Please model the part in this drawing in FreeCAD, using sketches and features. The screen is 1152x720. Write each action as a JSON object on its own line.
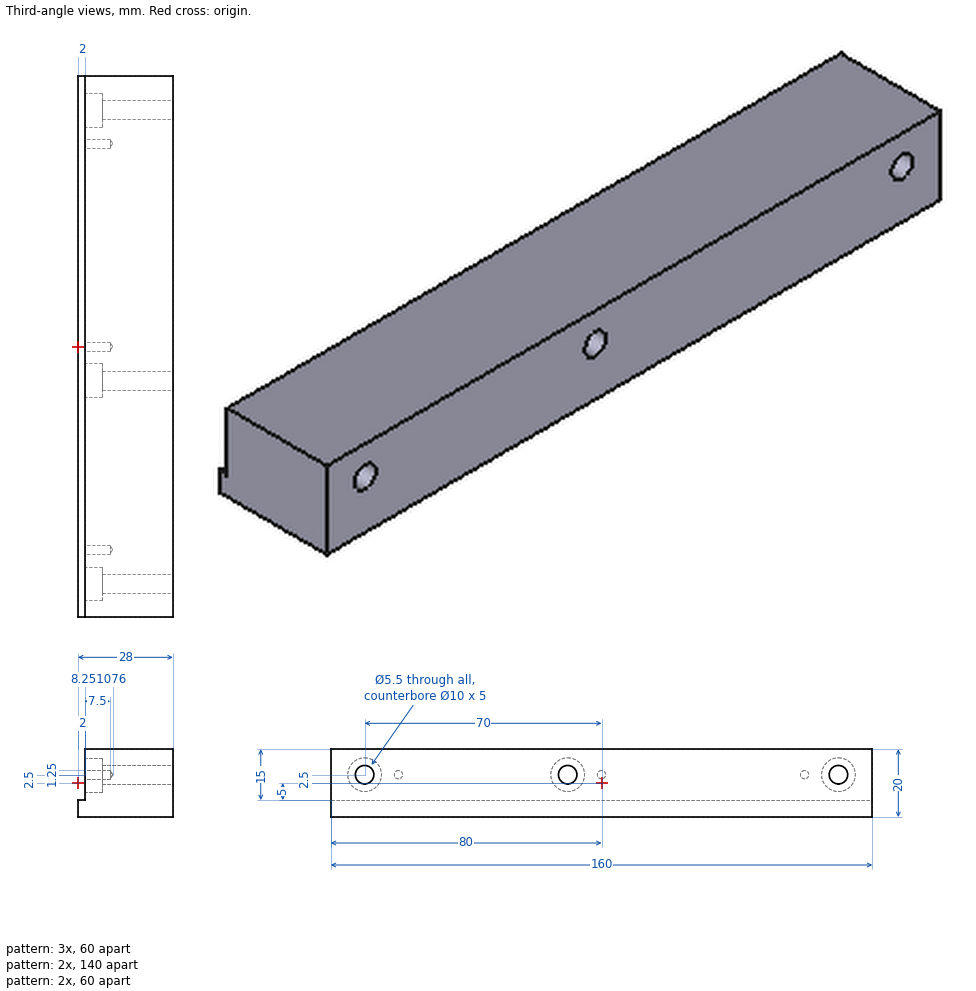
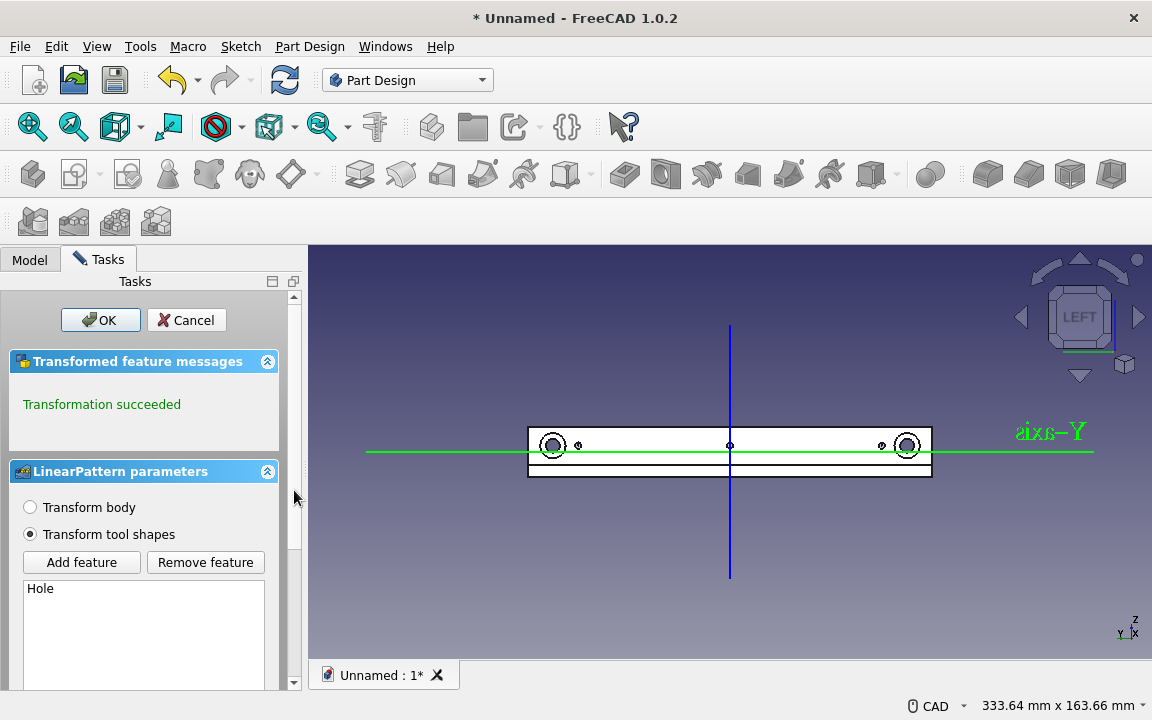
{"action": "left_click", "coordinate": [101, 320]}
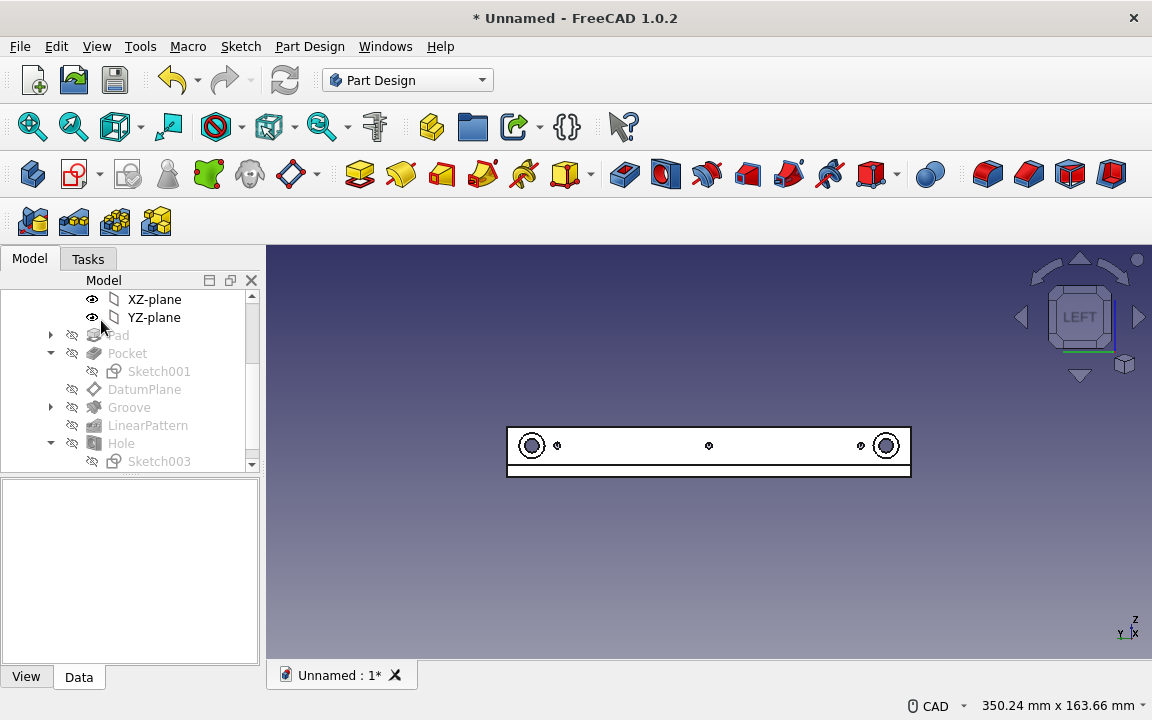
{"action": "left_click", "coordinate": [117, 443]}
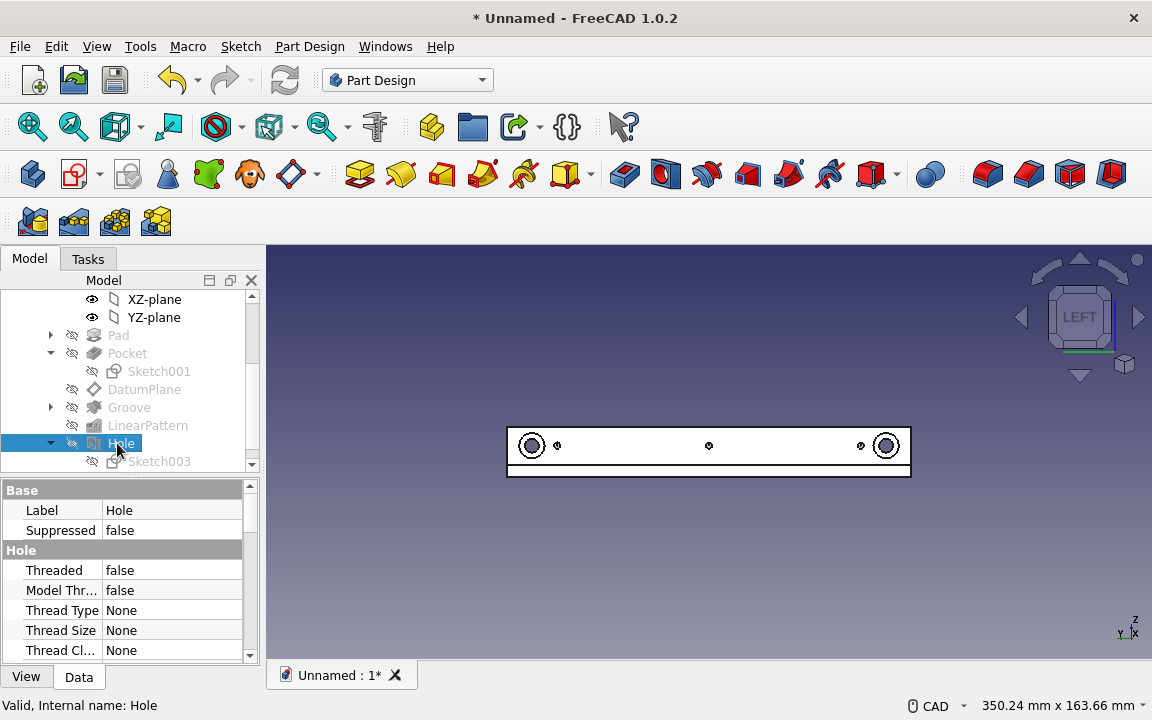
{"action": "left_click", "coordinate": [74, 222]}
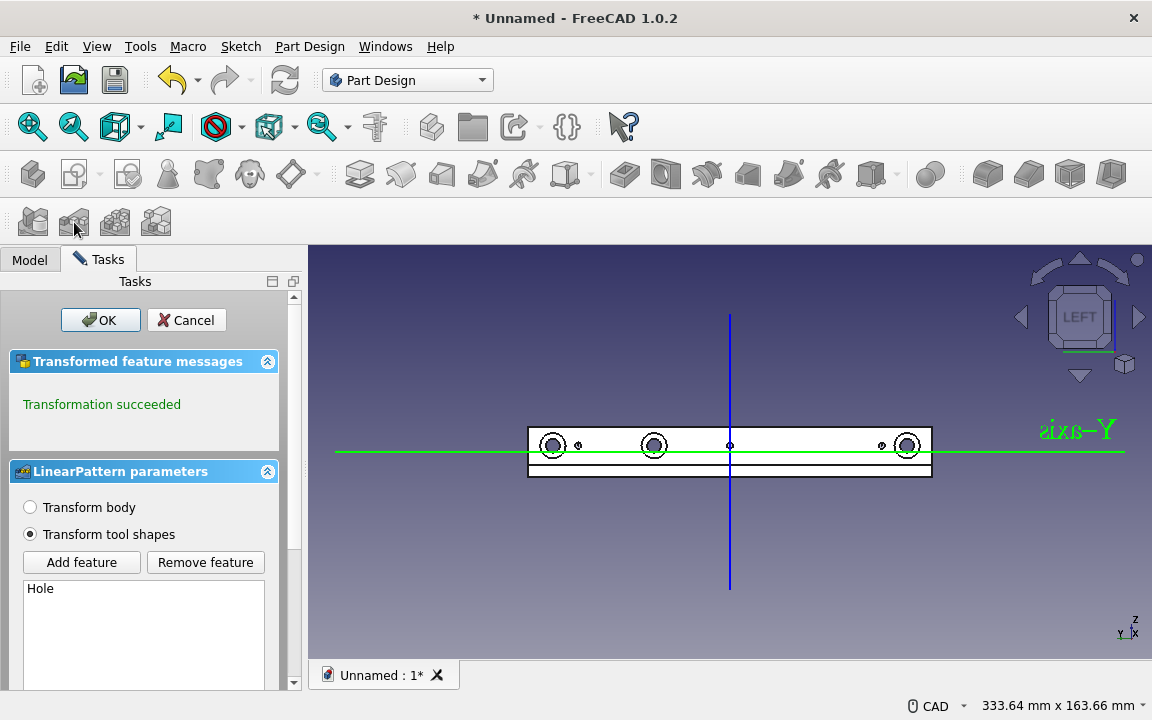
{"action": "scroll", "coordinate": [294, 490], "scroll_direction": "down", "scroll_amount": 2}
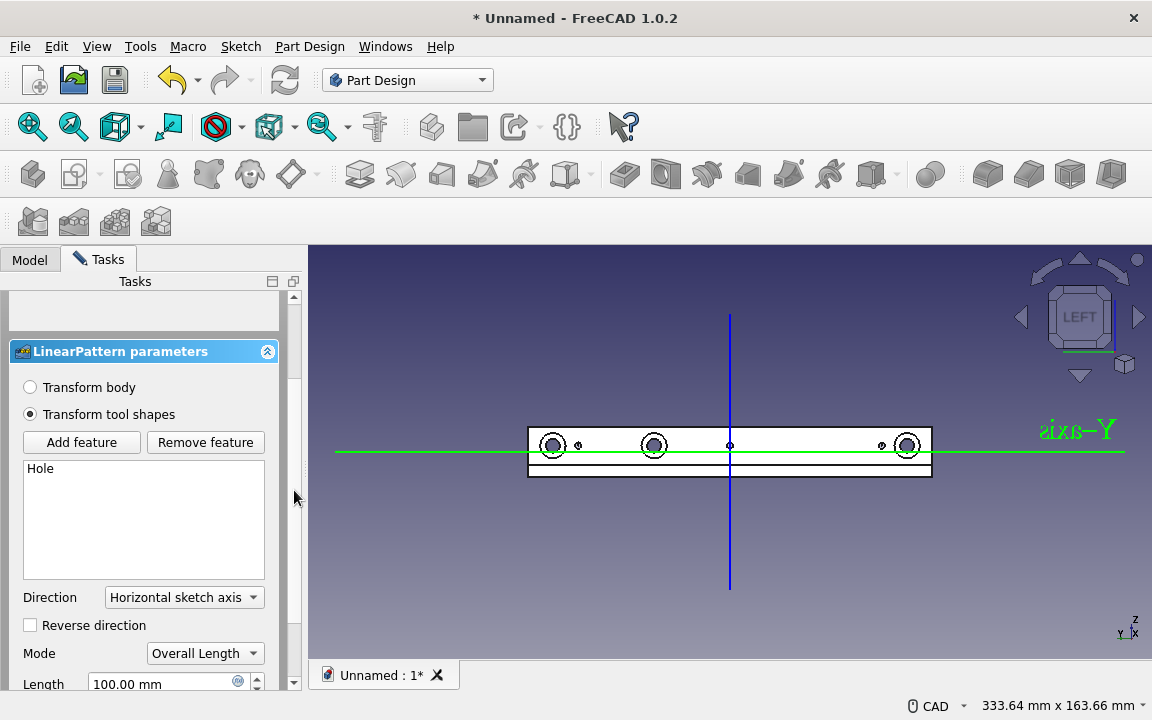
{"action": "left_click", "coordinate": [185, 598]}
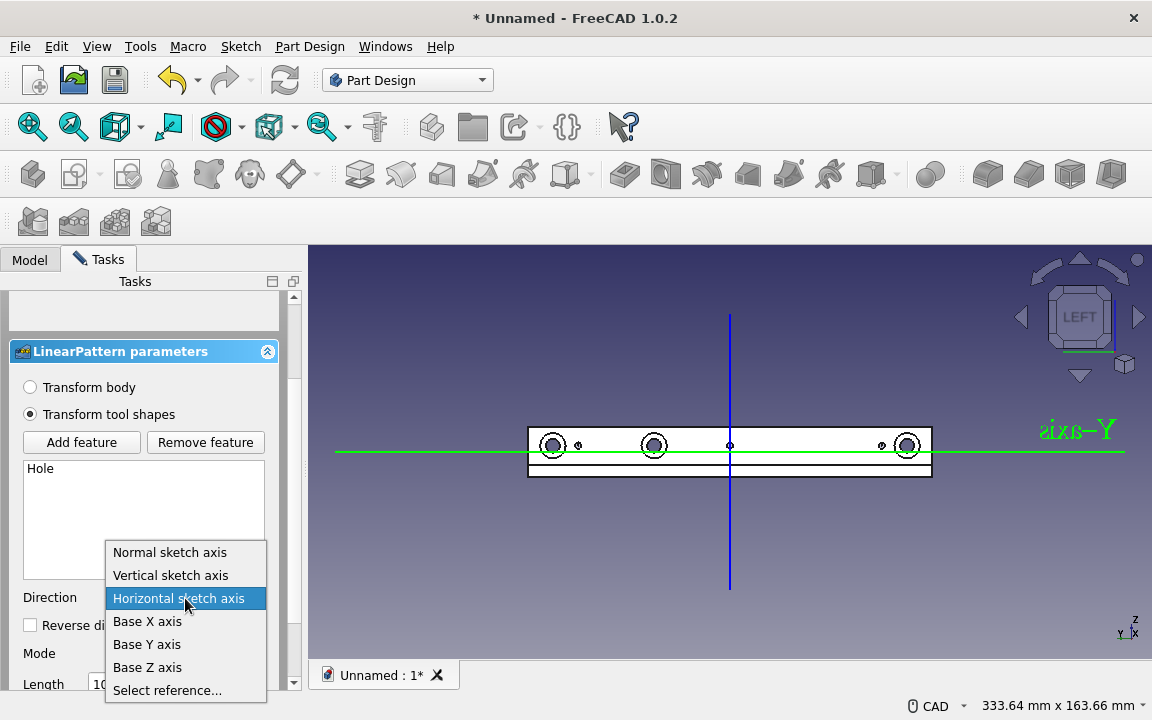
{"action": "left_click", "coordinate": [184, 644]}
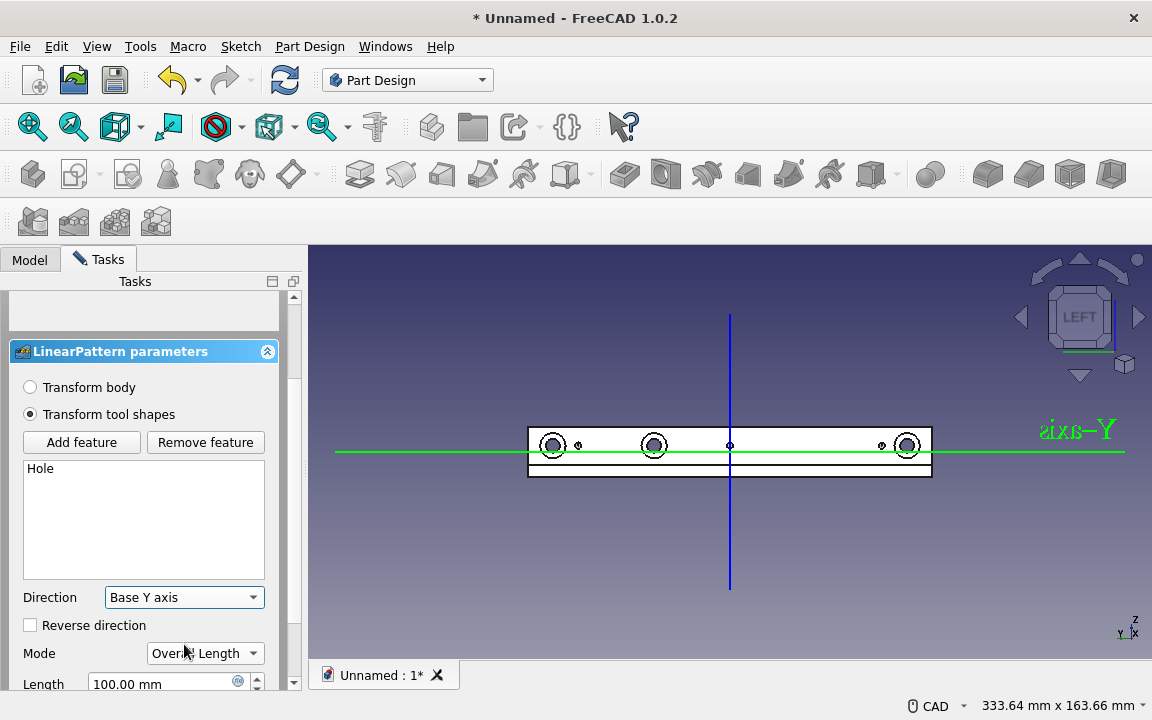
{"action": "left_click", "coordinate": [206, 654]}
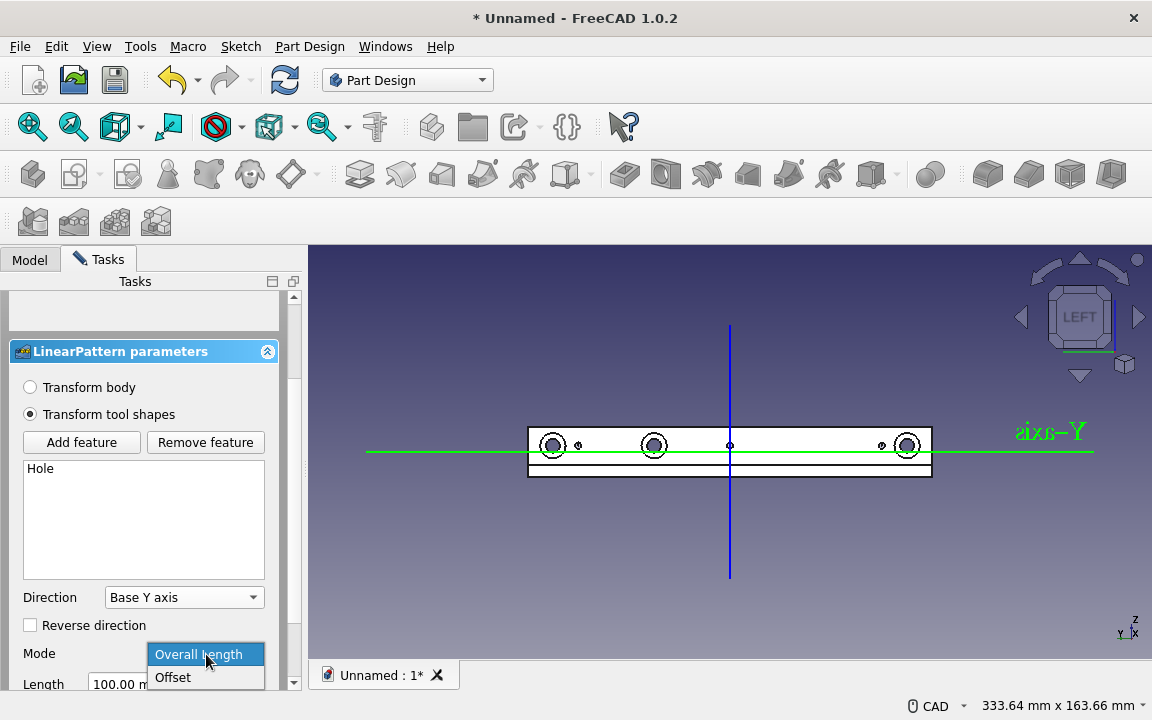
{"action": "left_click", "coordinate": [204, 678]}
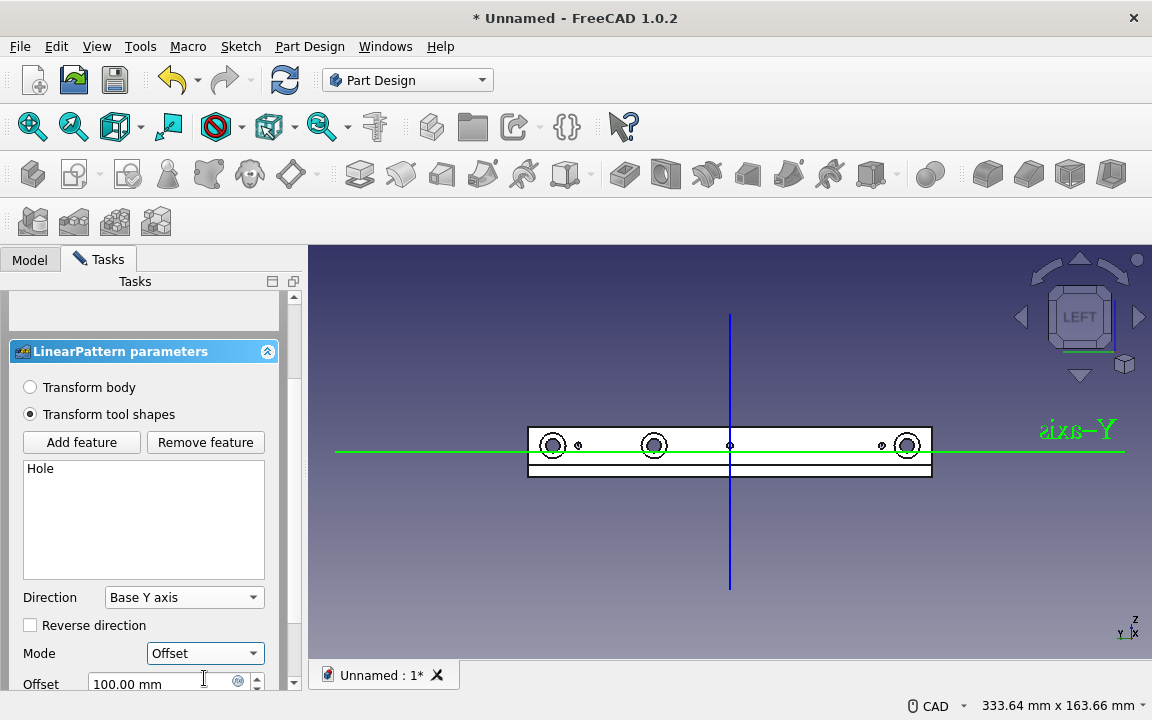
{"action": "scroll", "coordinate": [294, 490], "scroll_direction": "down", "scroll_amount": 2}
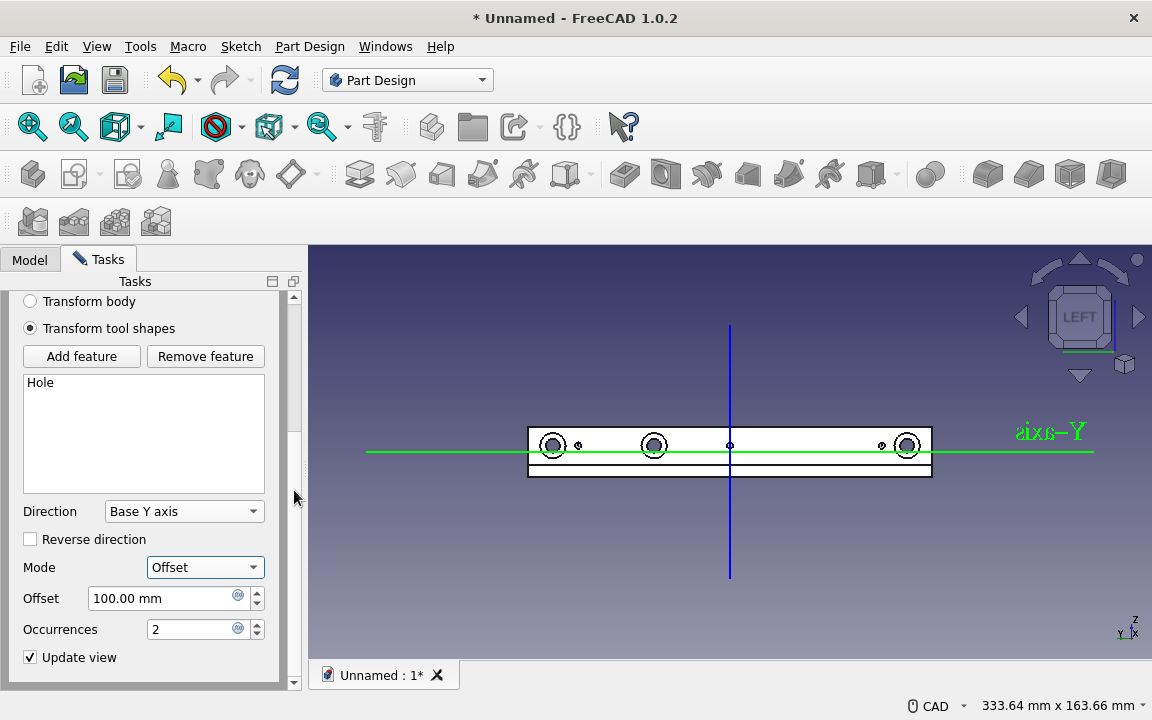
{"action": "triple_click", "coordinate": [170, 598]}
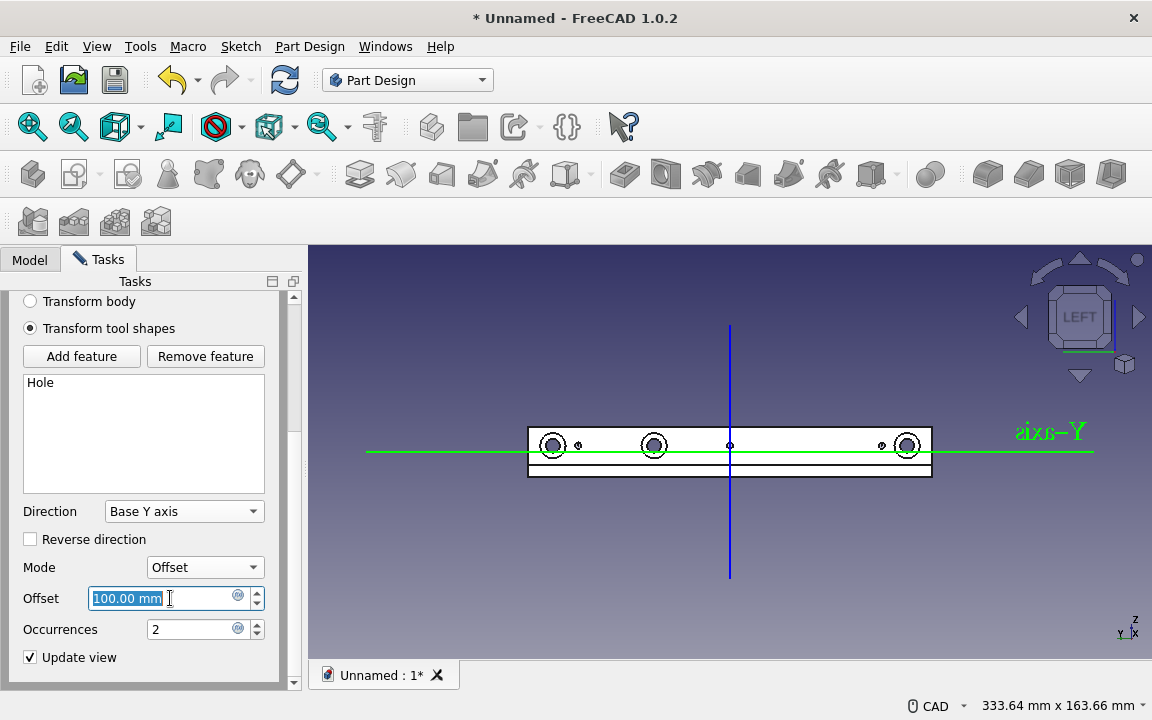
{"action": "type", "text": "60"}
{"action": "key", "text": "Tab"}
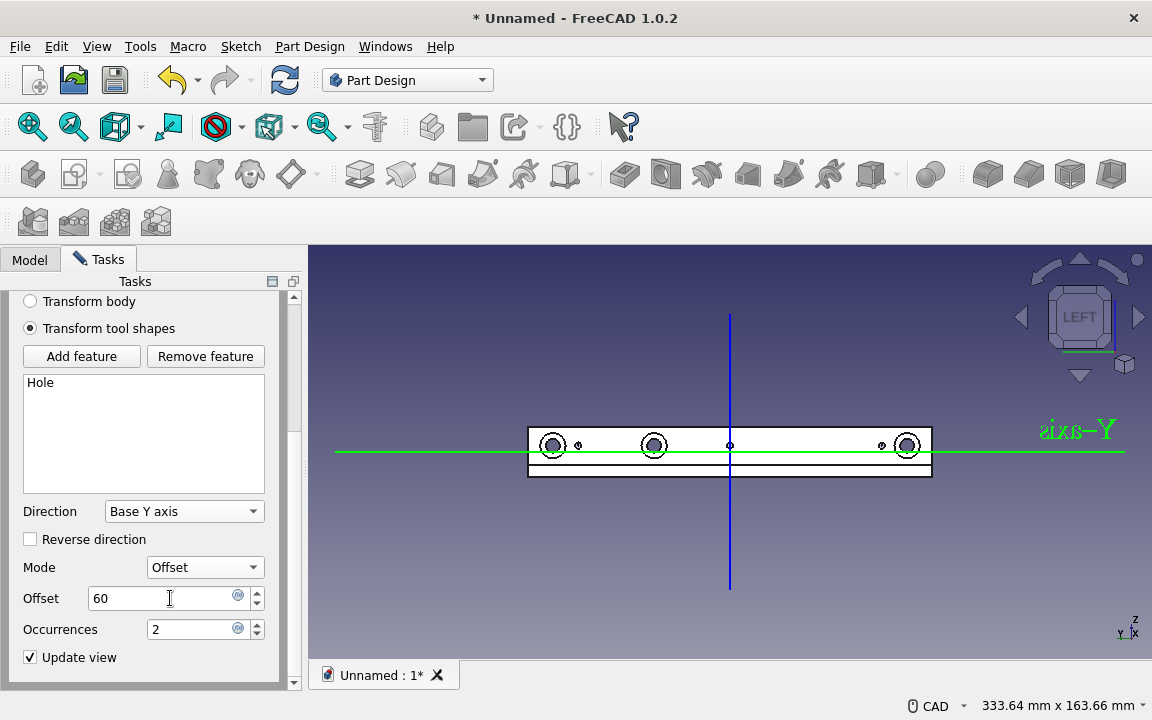
{"action": "triple_click", "coordinate": [199, 630]}